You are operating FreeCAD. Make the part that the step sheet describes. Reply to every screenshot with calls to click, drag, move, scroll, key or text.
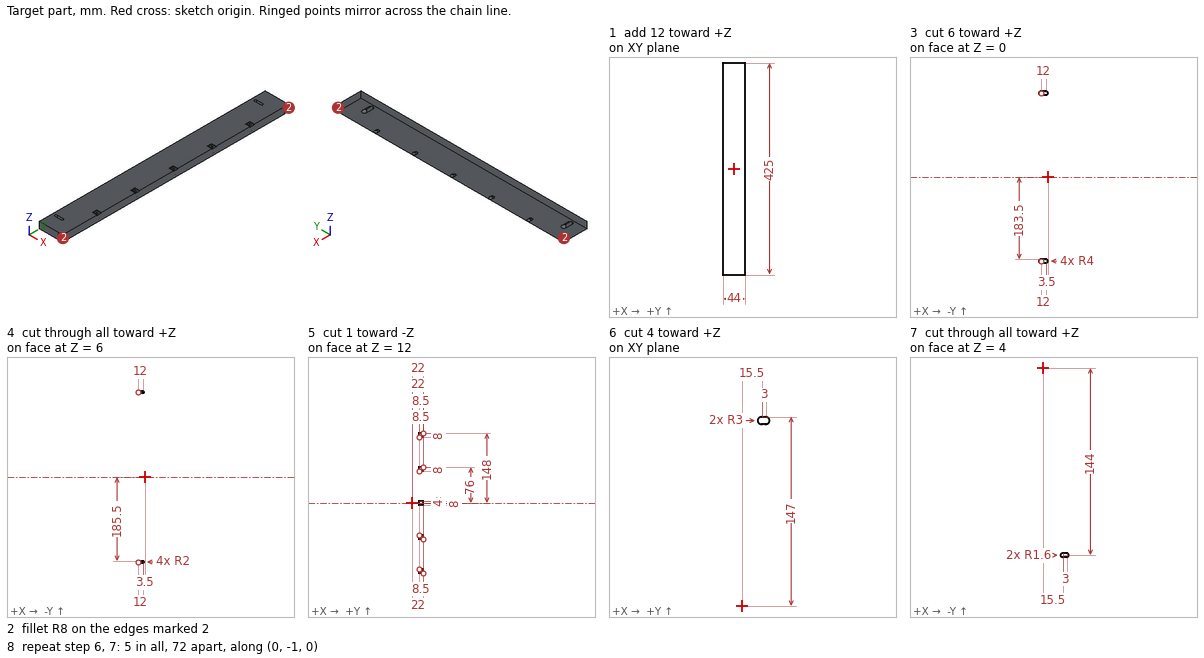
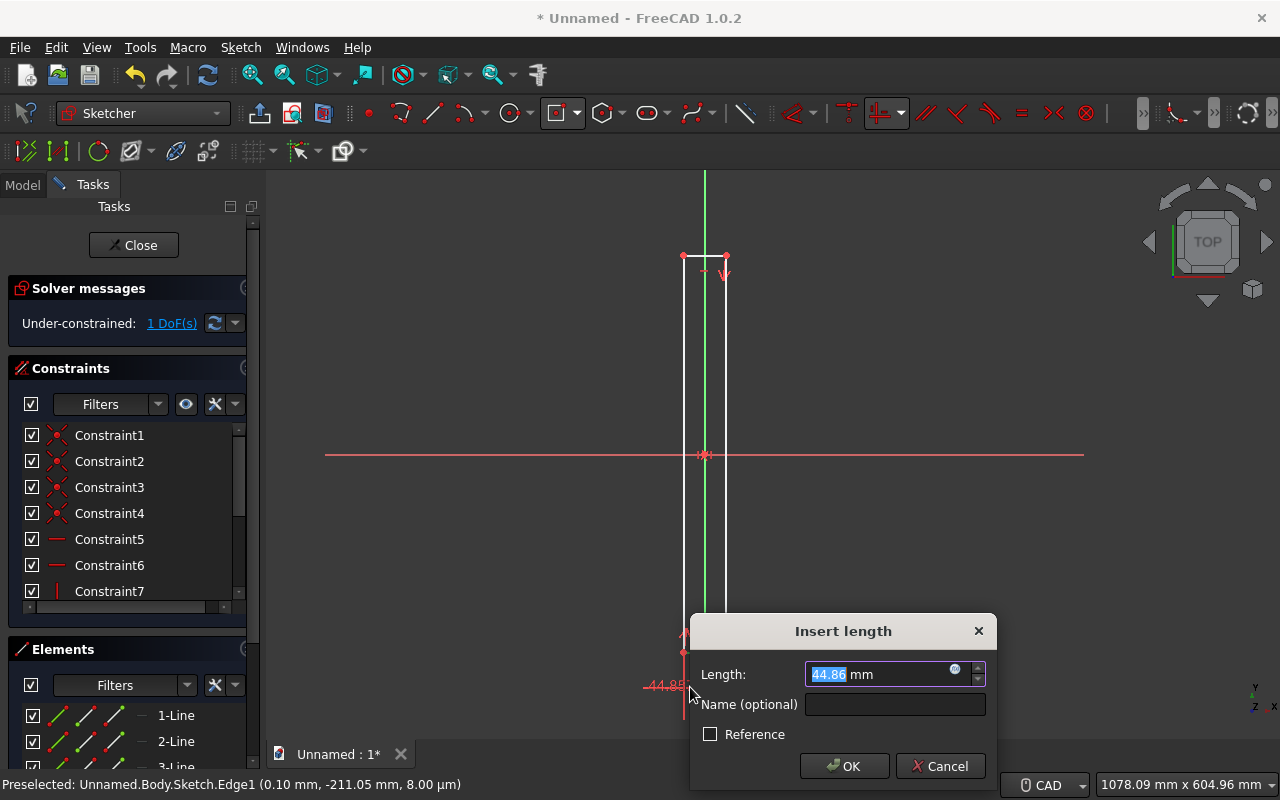
text(44)
key(Return)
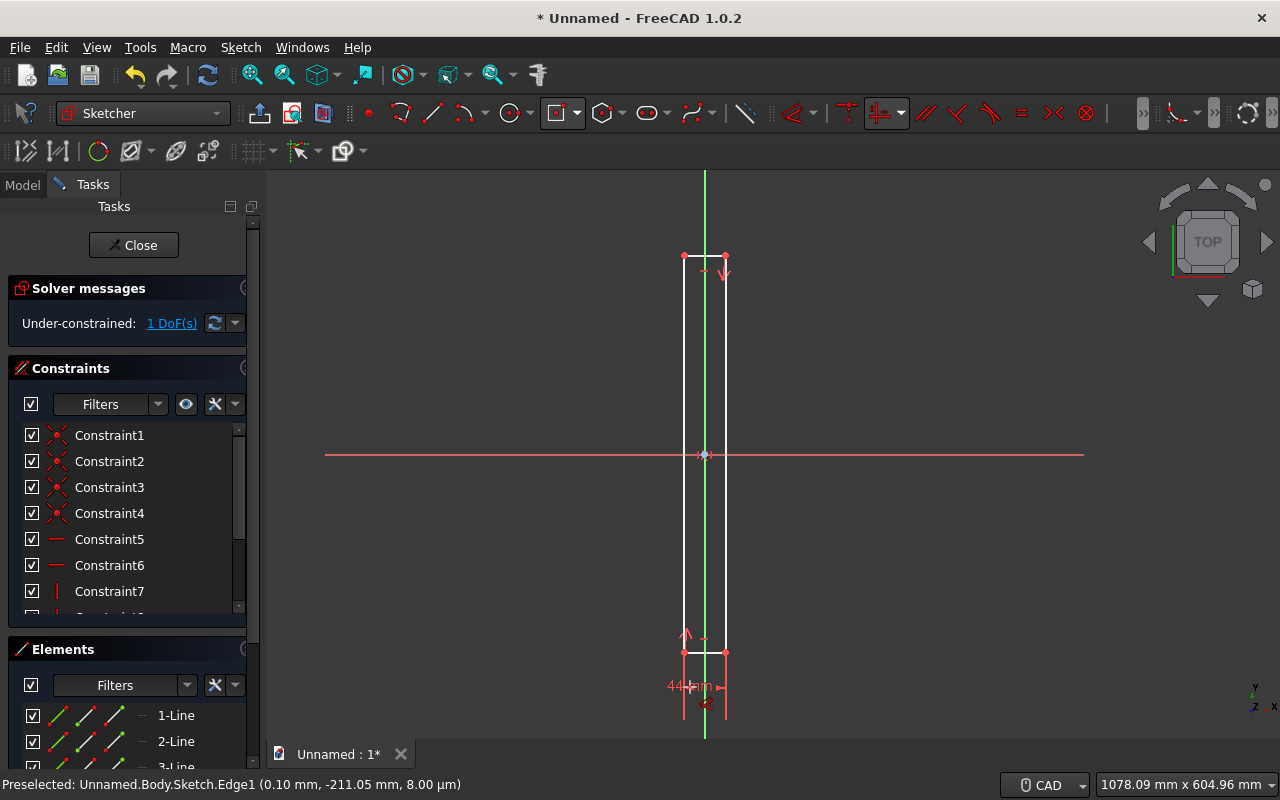
click(726, 534)
click(760, 363)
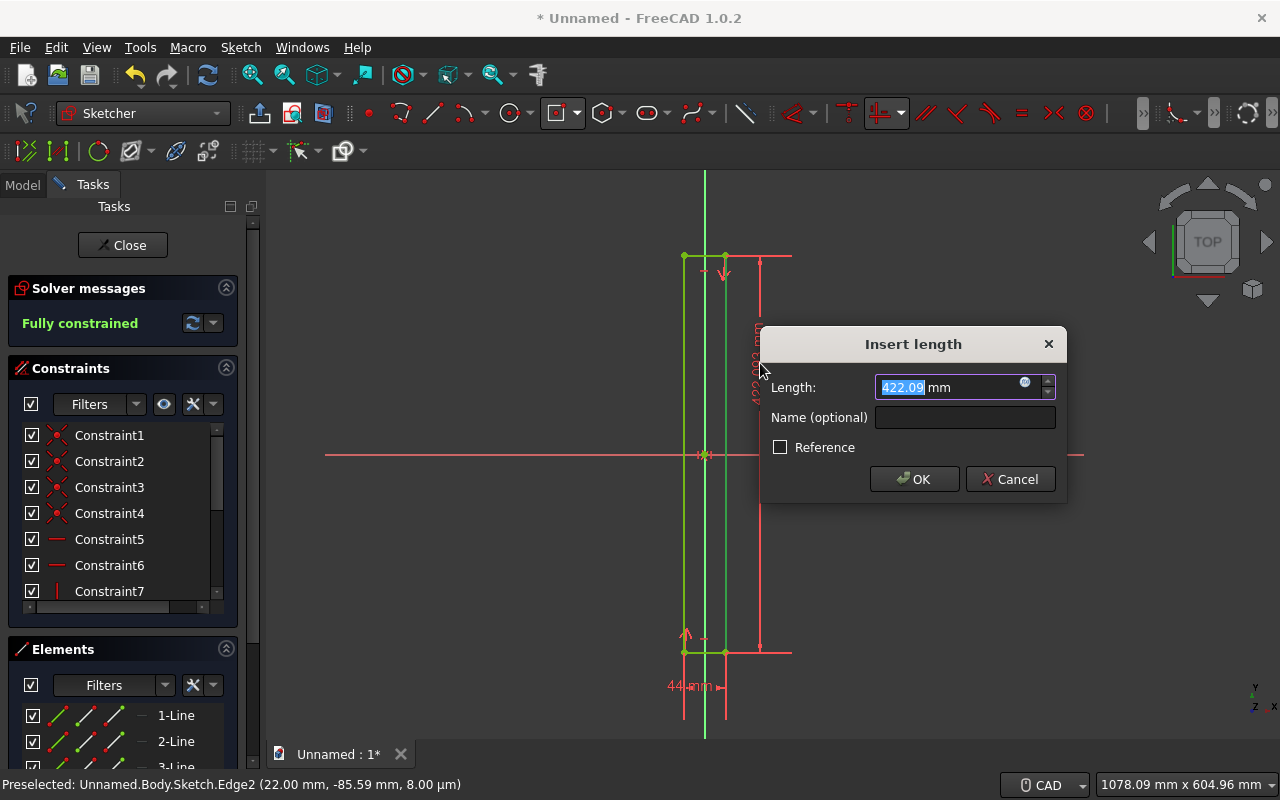
text(425)
key(Return)
key(Escape)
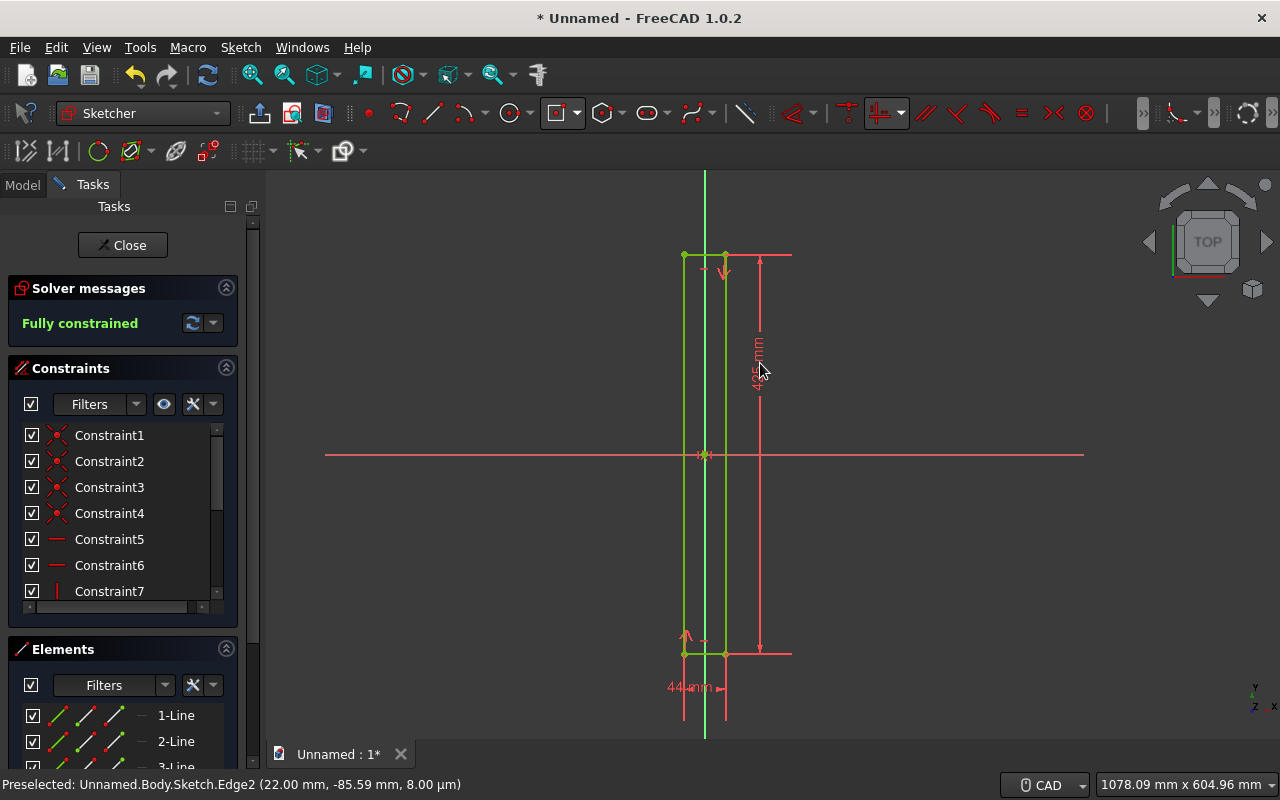
click(123, 245)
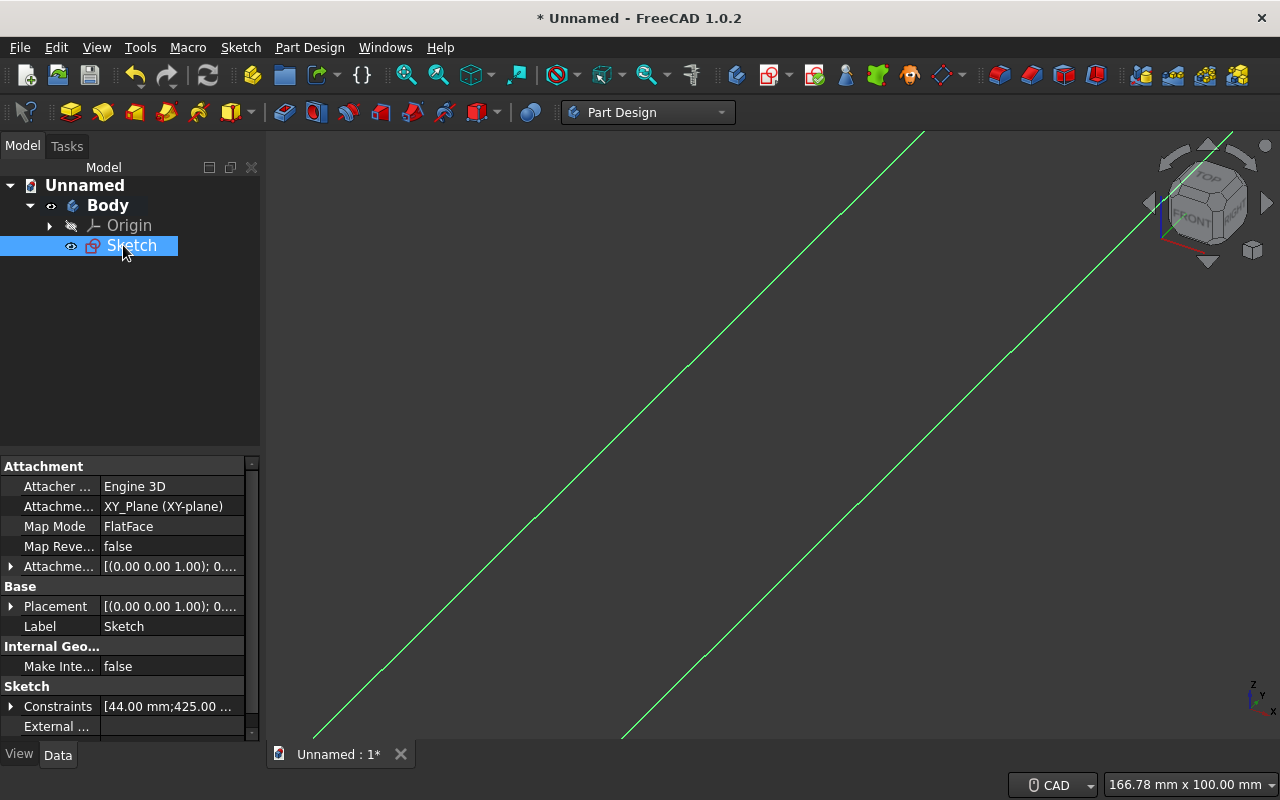
click(72, 112)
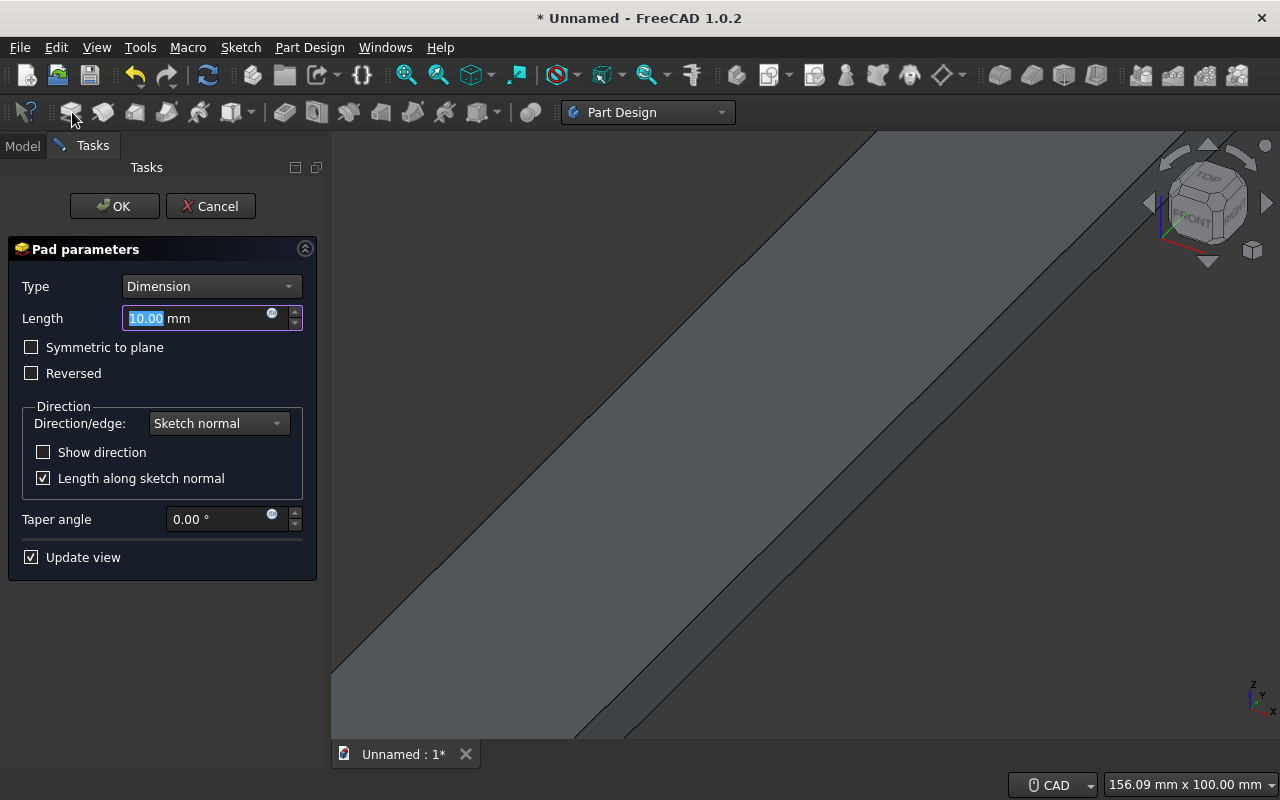
text(12)
key(Tab)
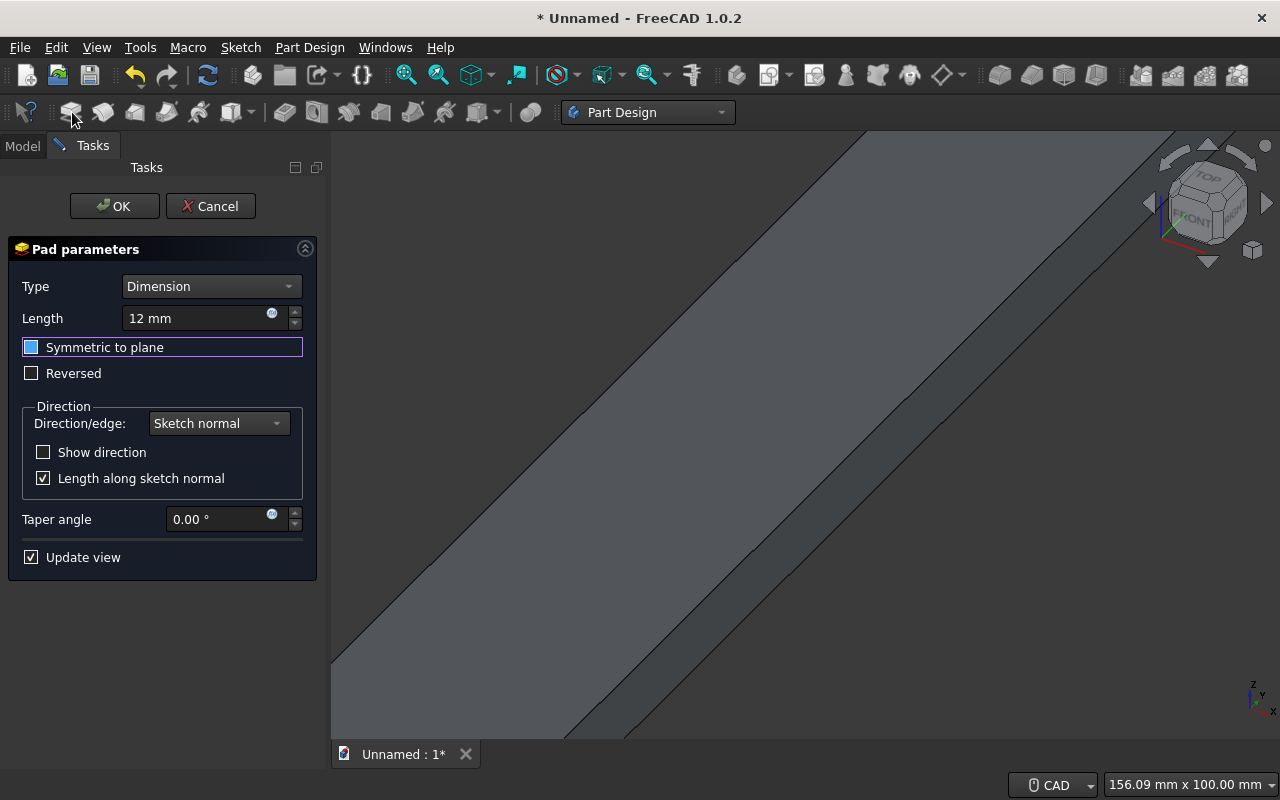
click(115, 206)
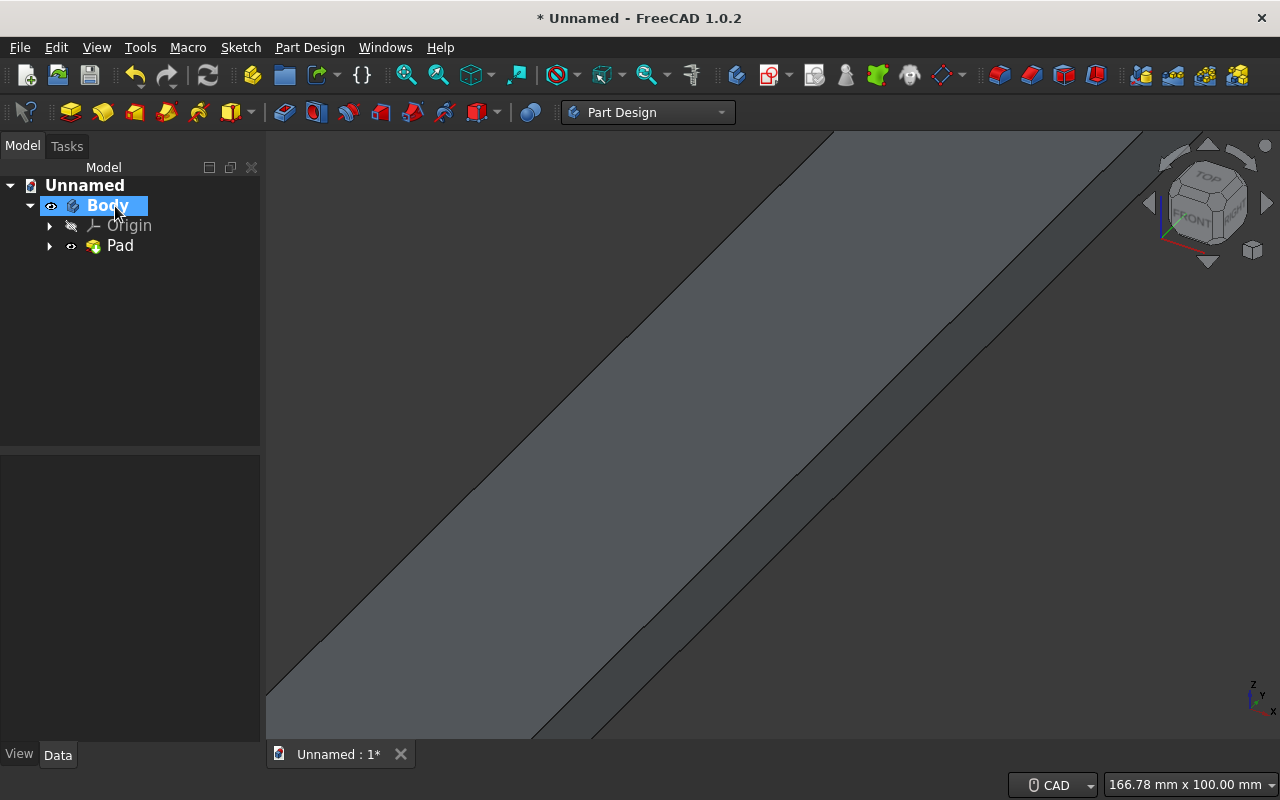
click(408, 76)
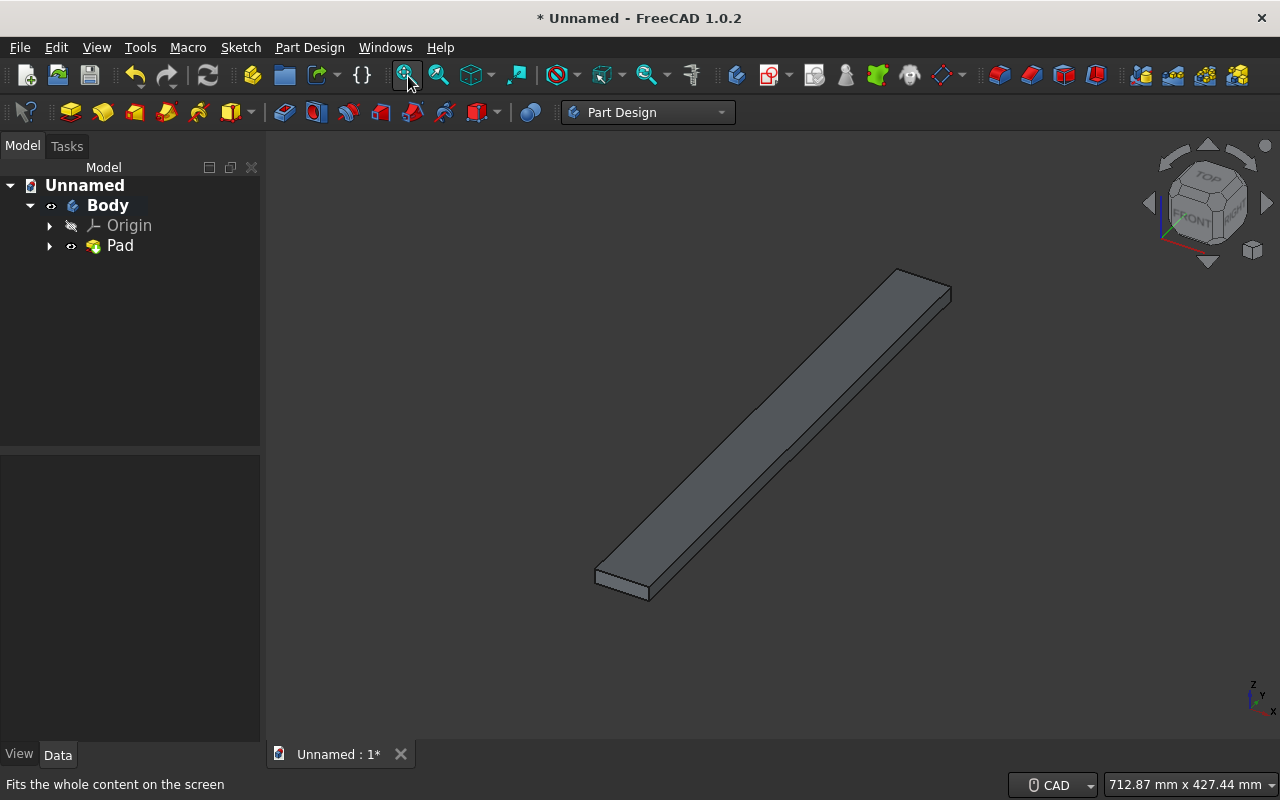
click(649, 593)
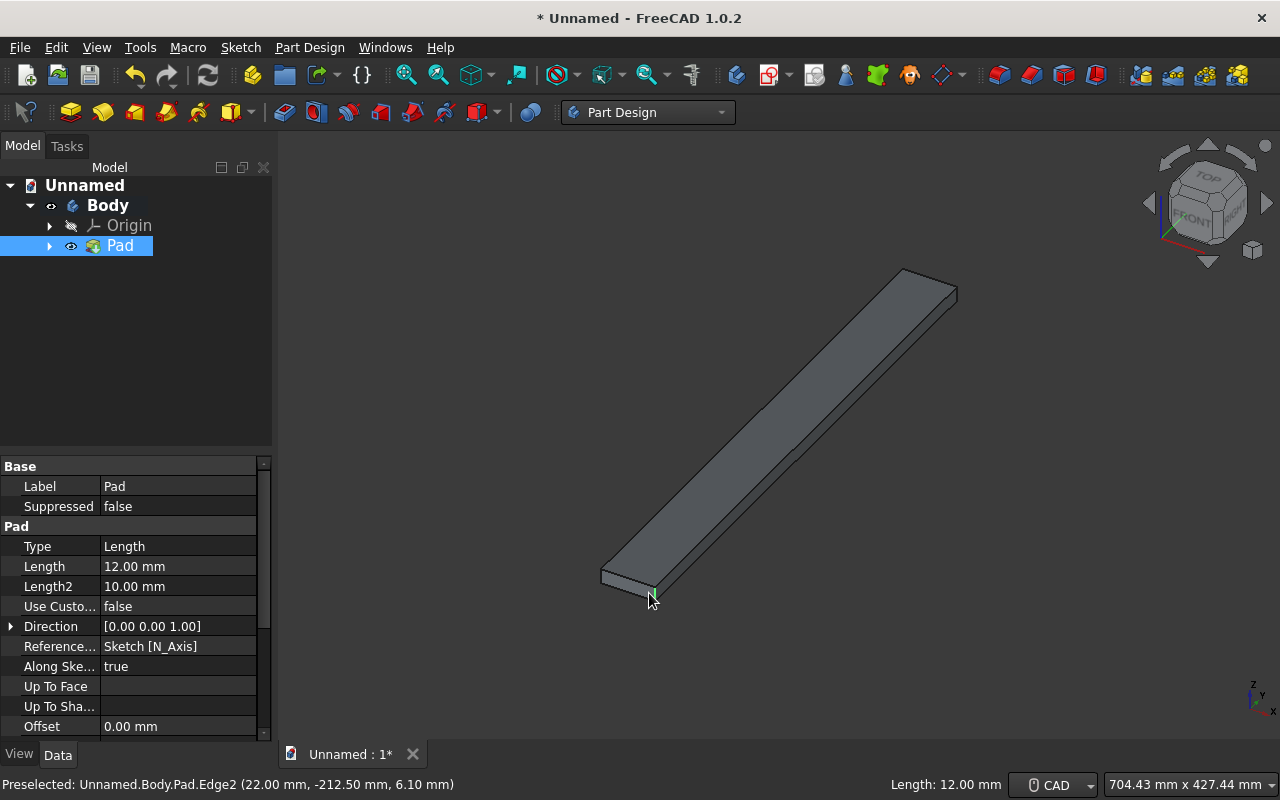
scroll(957, 293, up, 5)